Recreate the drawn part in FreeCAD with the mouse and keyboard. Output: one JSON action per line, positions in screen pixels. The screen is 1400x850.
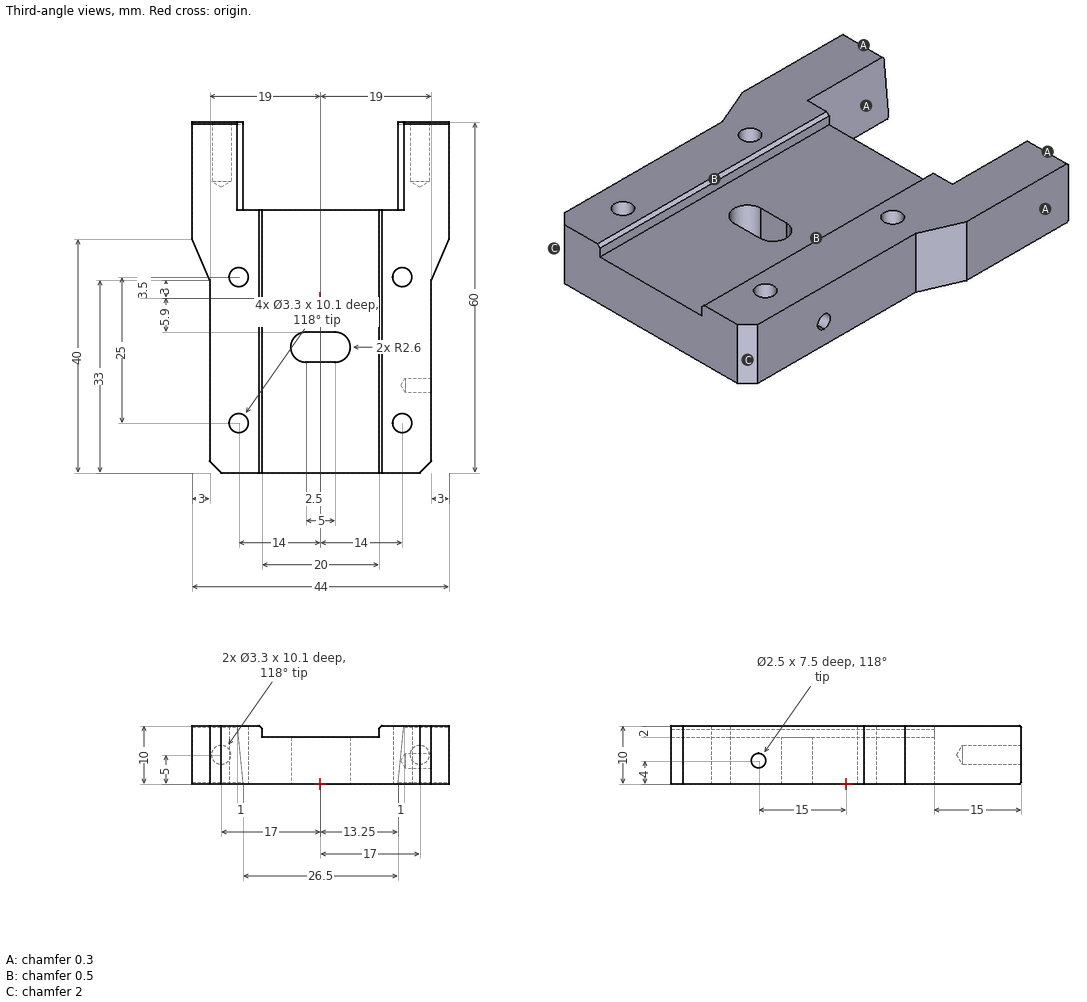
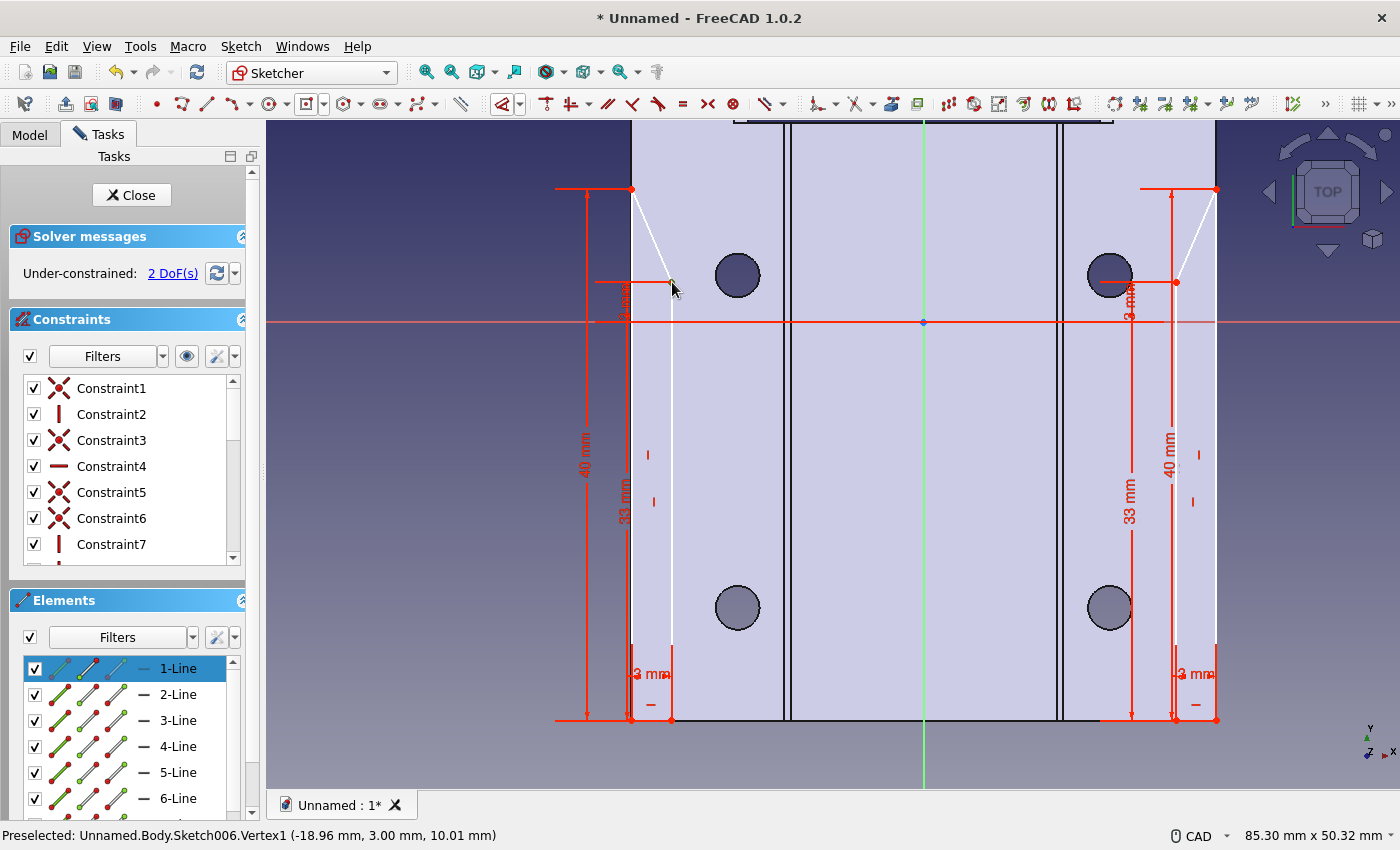
{"action": "left_click", "coordinate": [520, 104]}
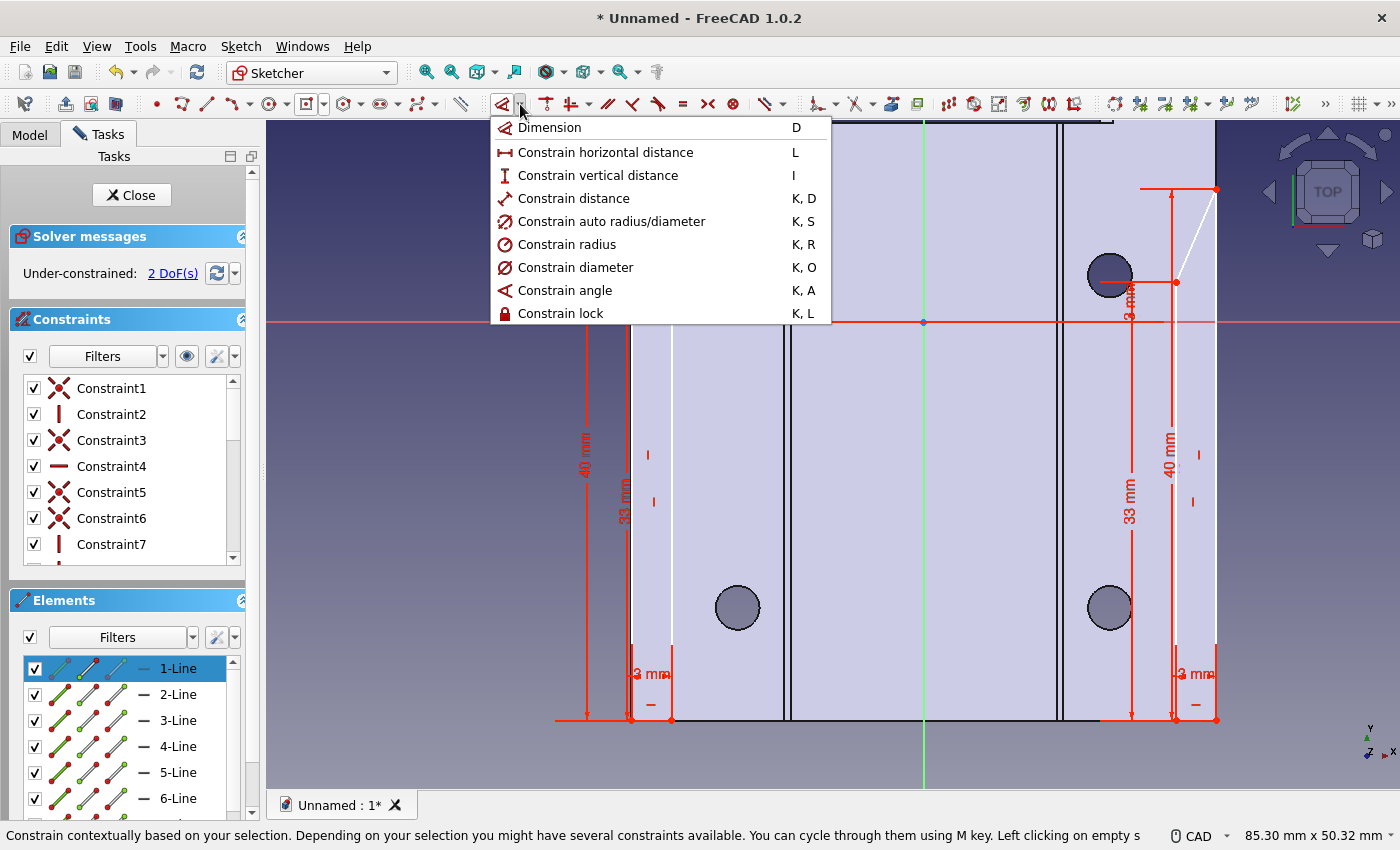
{"action": "left_click", "coordinate": [661, 152]}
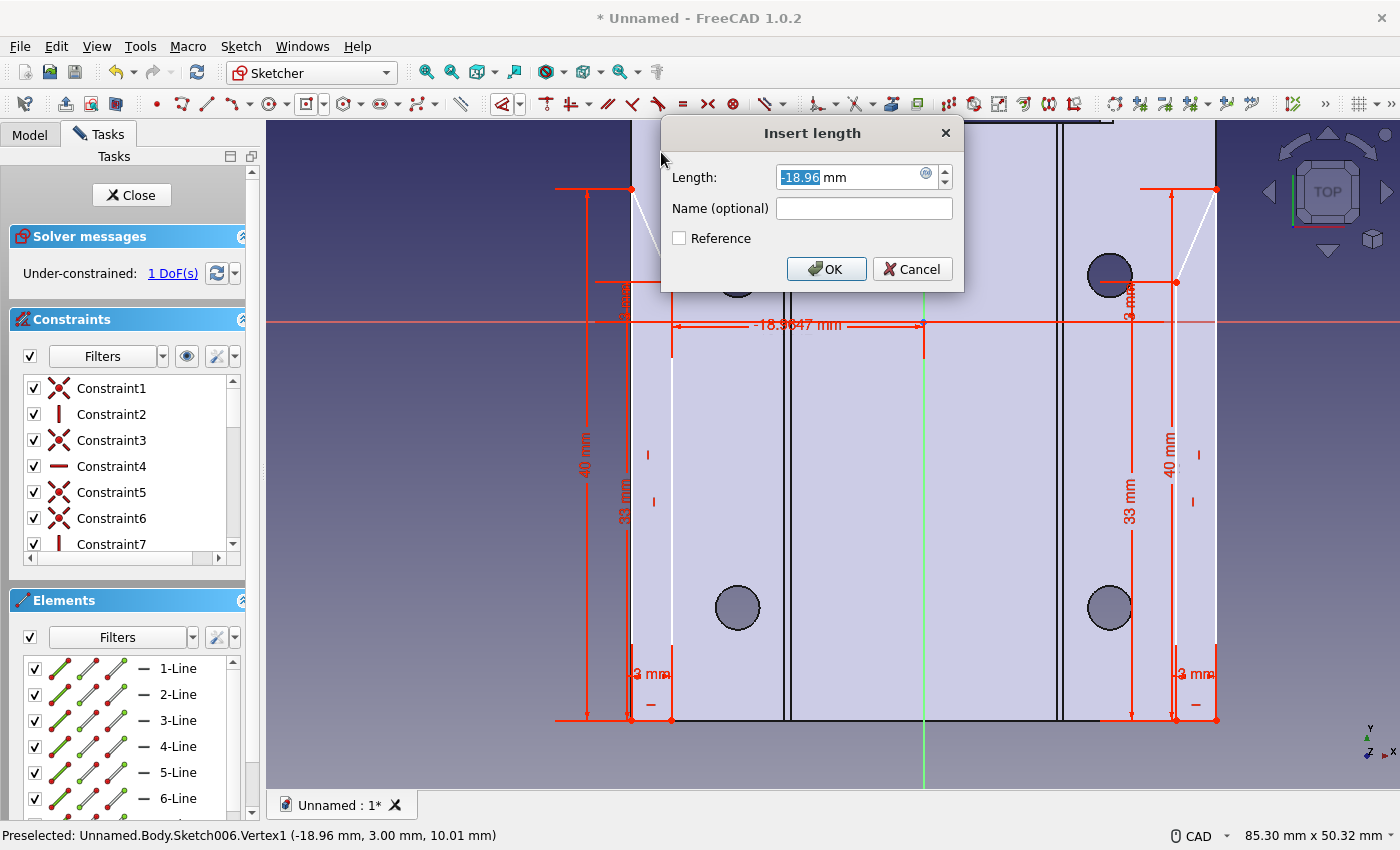
{"action": "type", "text": "-19"}
{"action": "key", "text": "Return"}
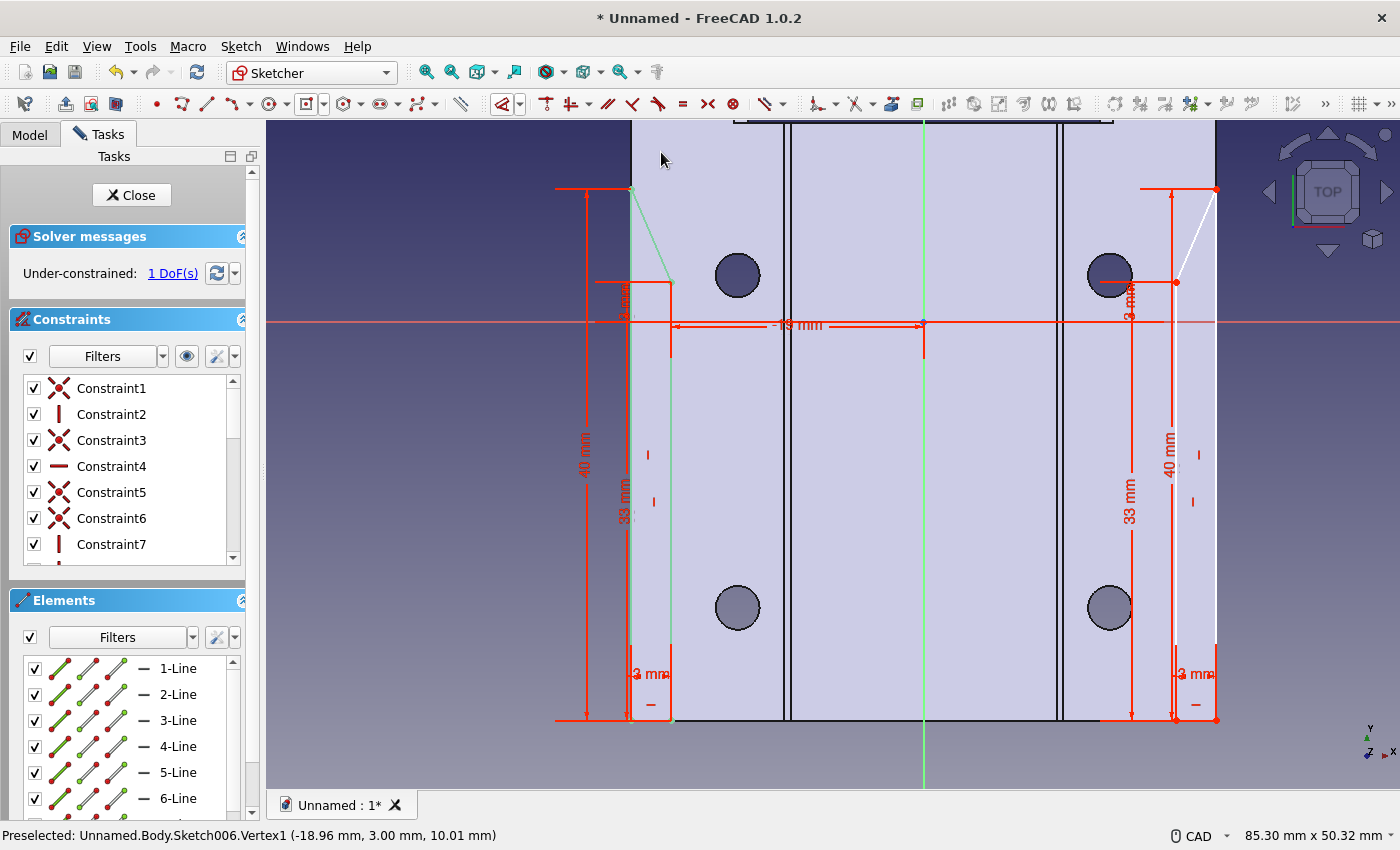
{"action": "left_click", "coordinate": [1176, 282]}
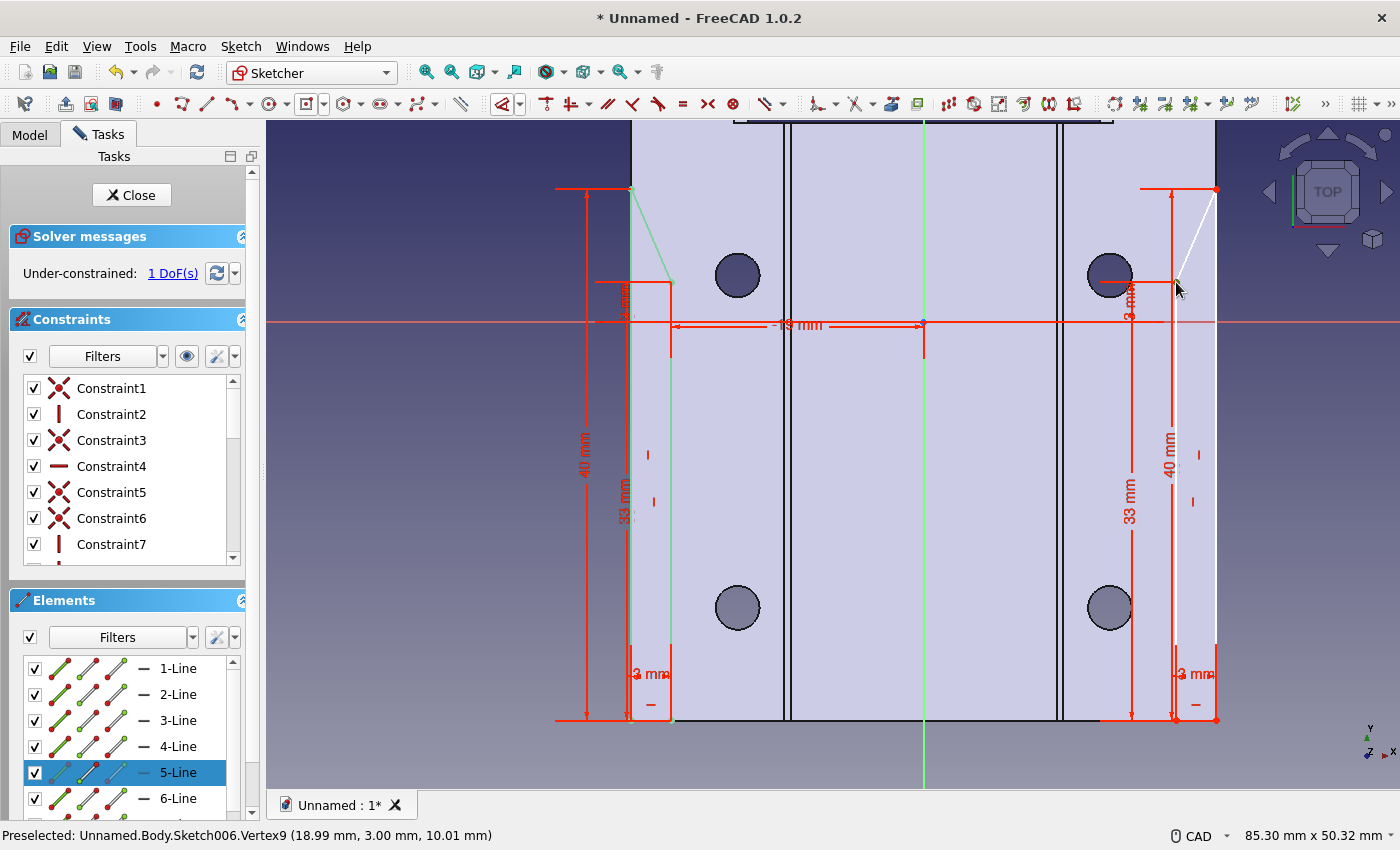
{"action": "left_click", "coordinate": [520, 104]}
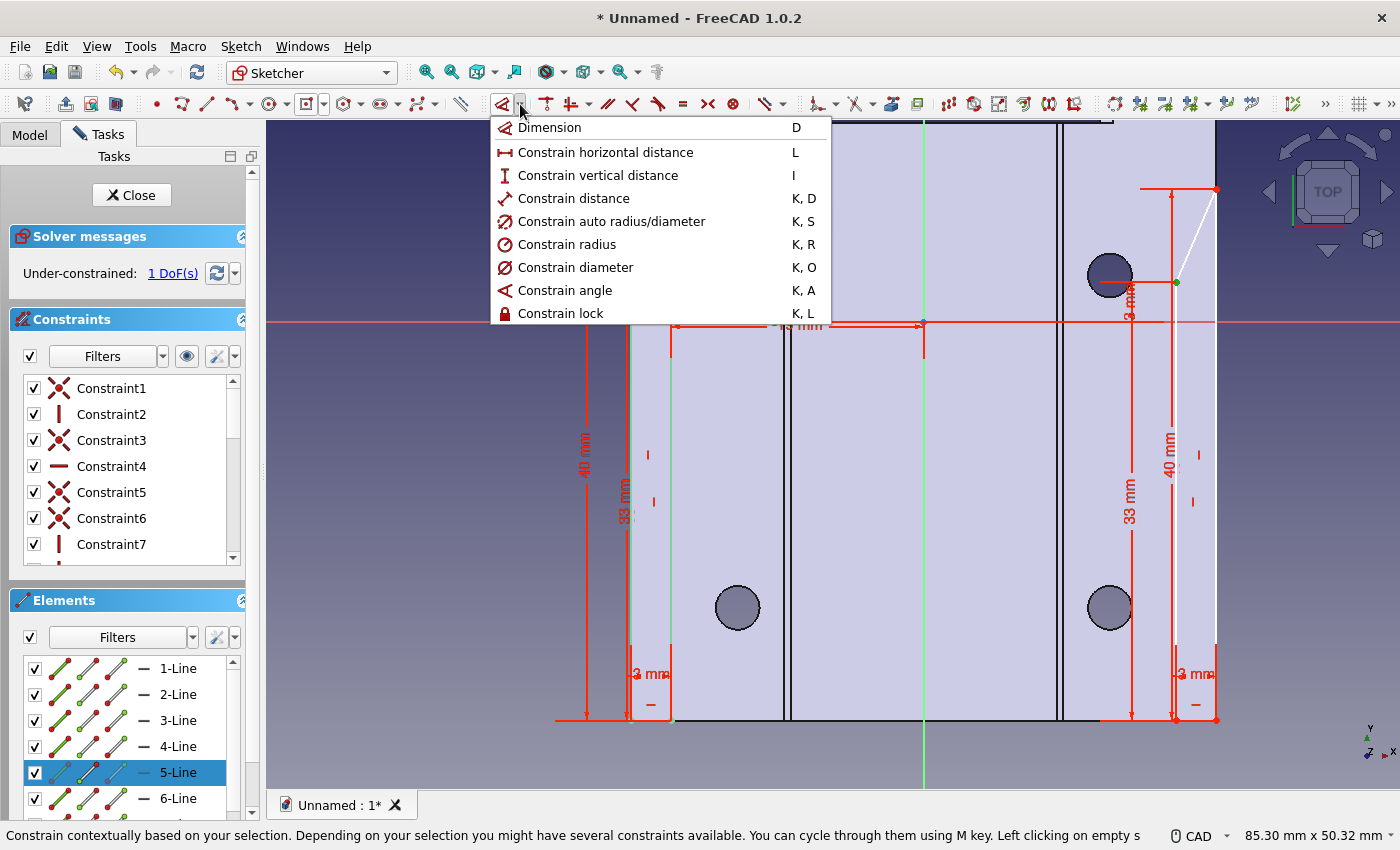
{"action": "left_click", "coordinate": [661, 152]}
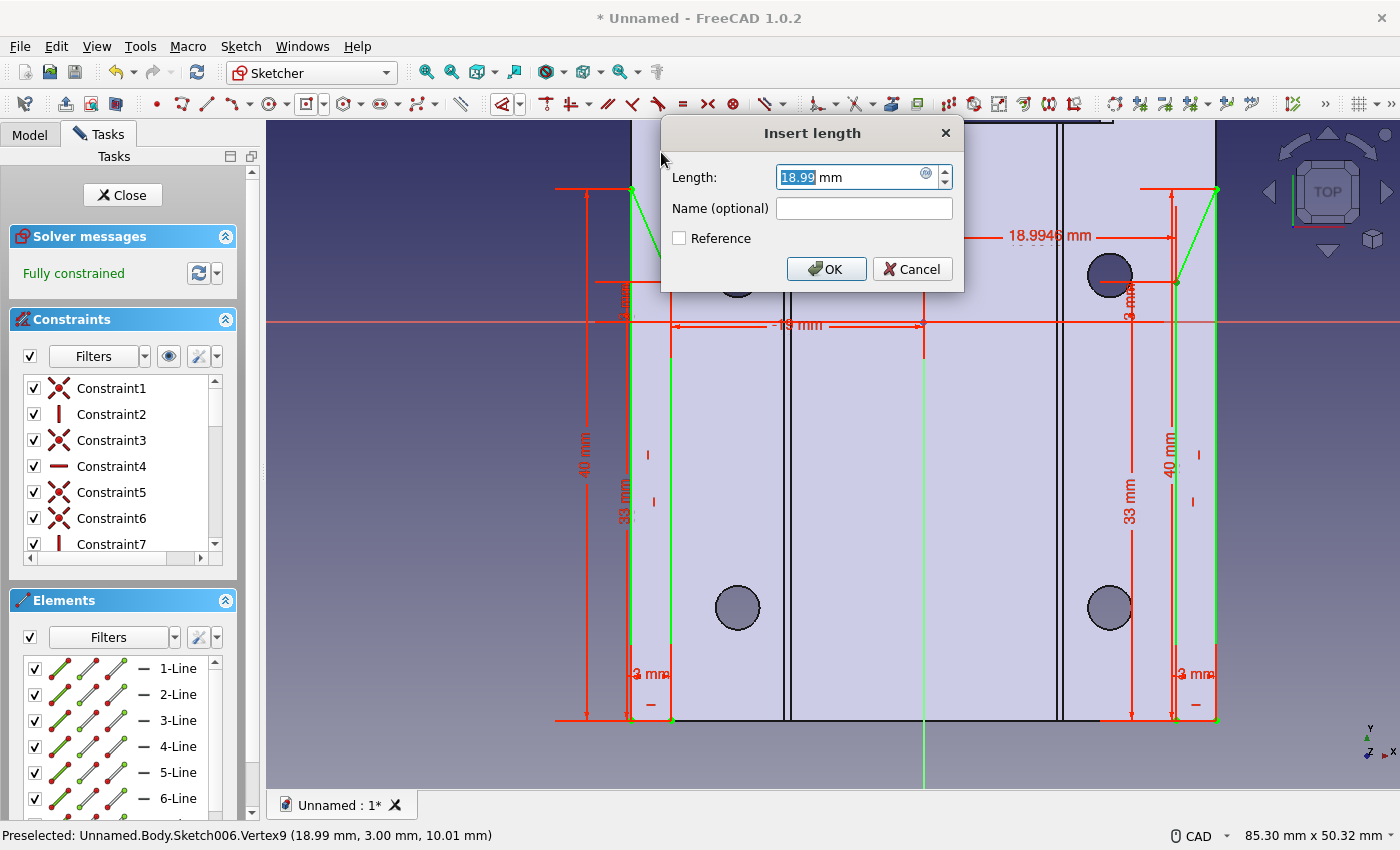
{"action": "type", "text": "19"}
{"action": "key", "text": "Return"}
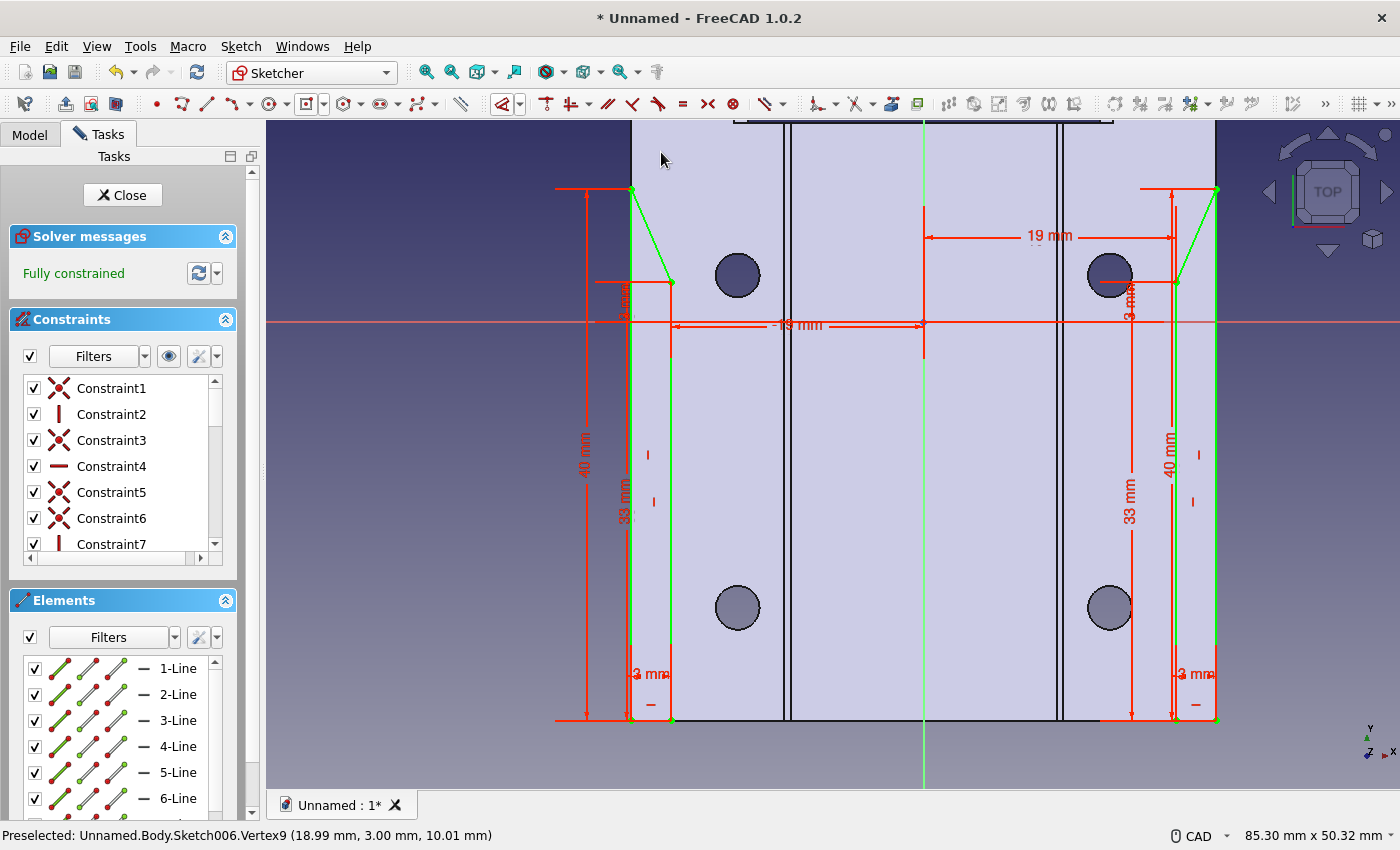
{"action": "left_click", "coordinate": [123, 195]}